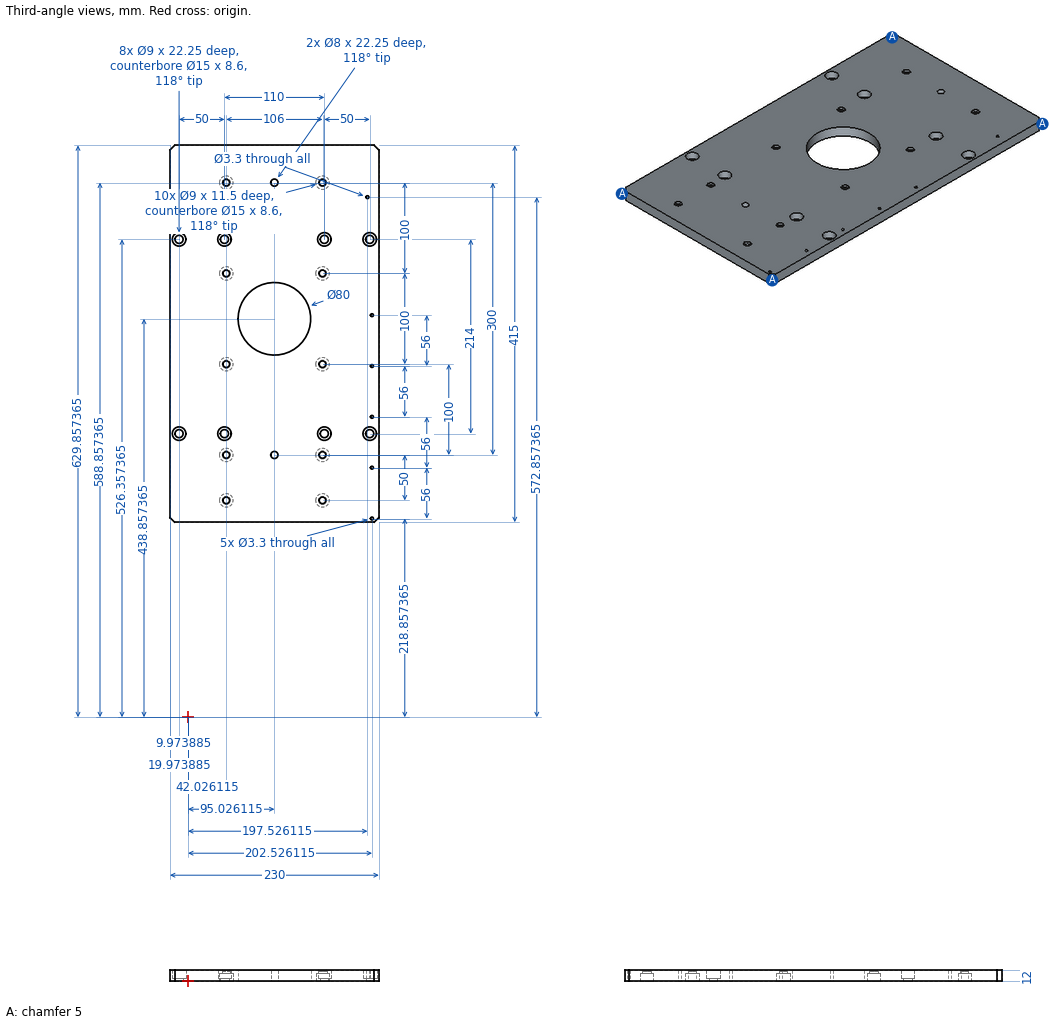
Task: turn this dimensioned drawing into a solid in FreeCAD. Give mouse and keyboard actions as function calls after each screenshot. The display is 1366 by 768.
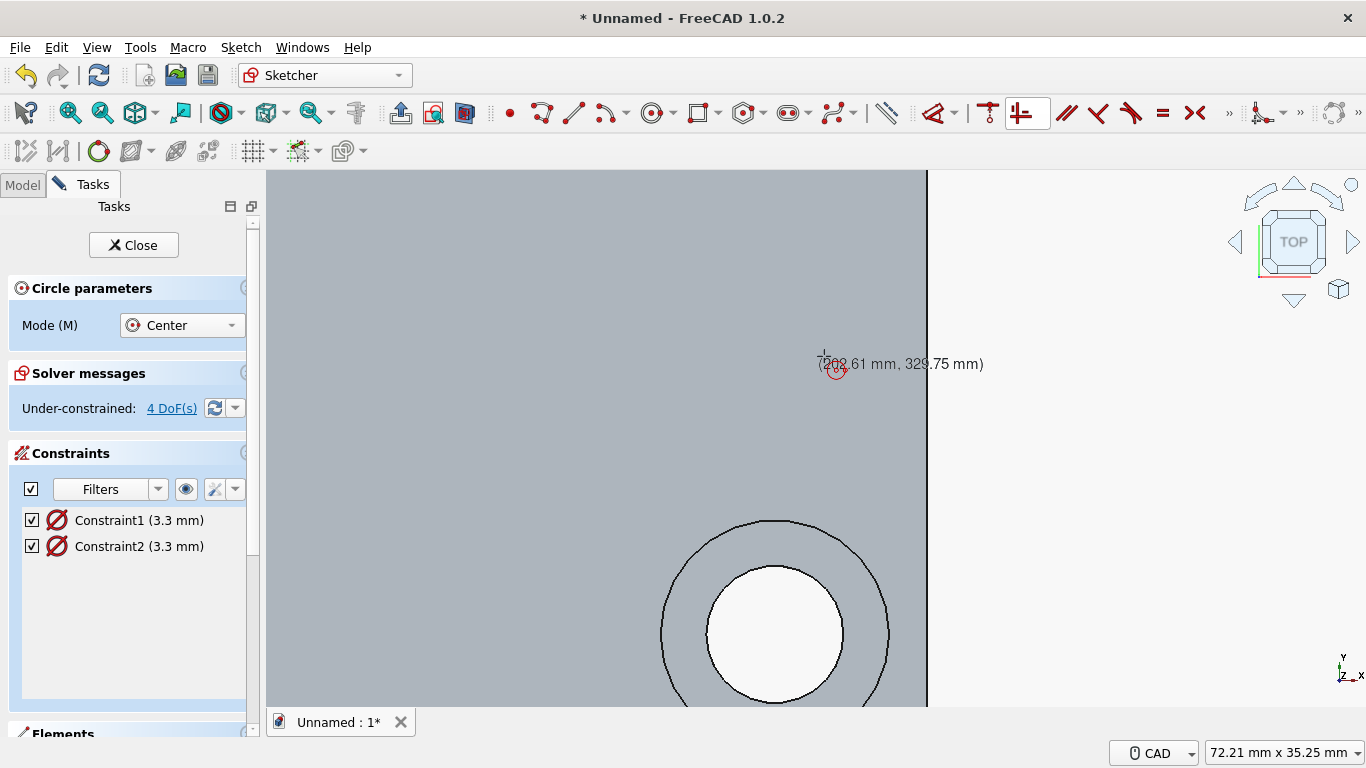
scroll(824, 356, down, 15)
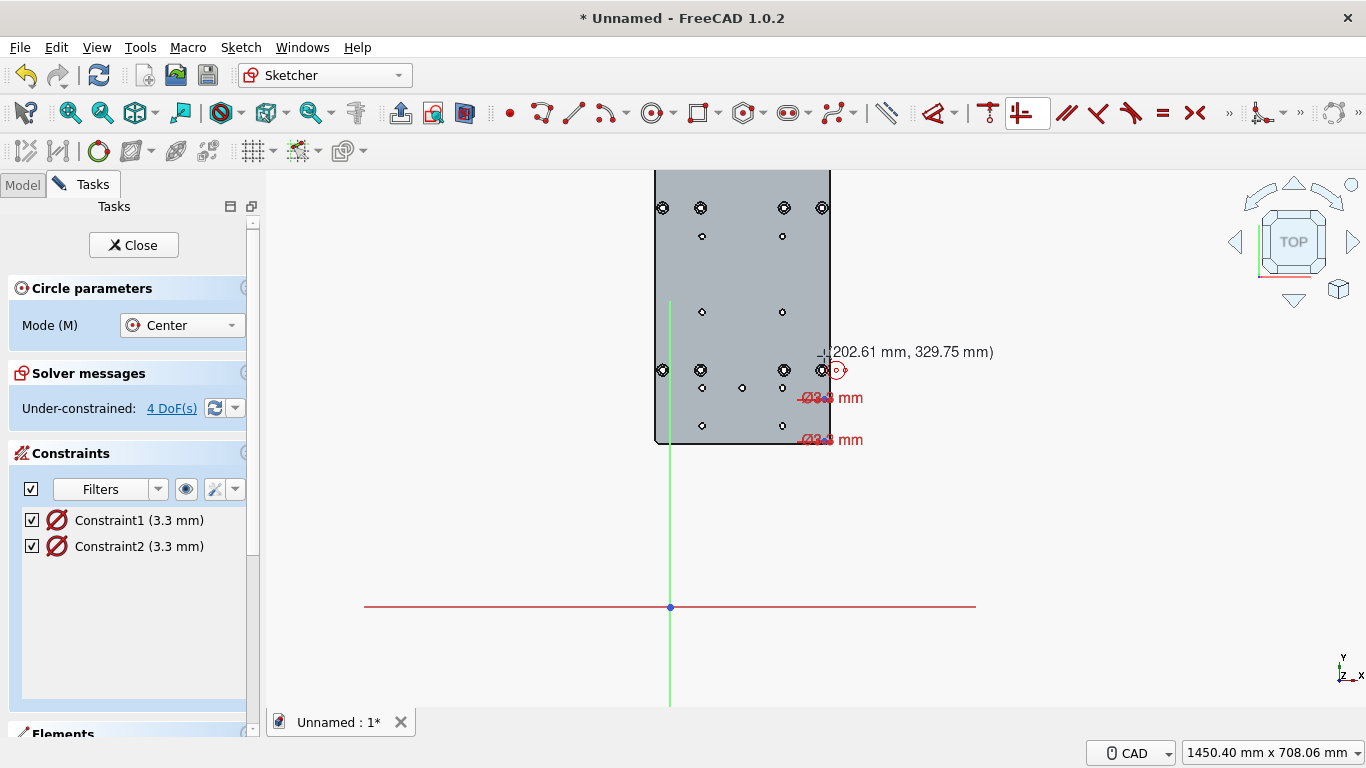
click(824, 356)
move(825, 355)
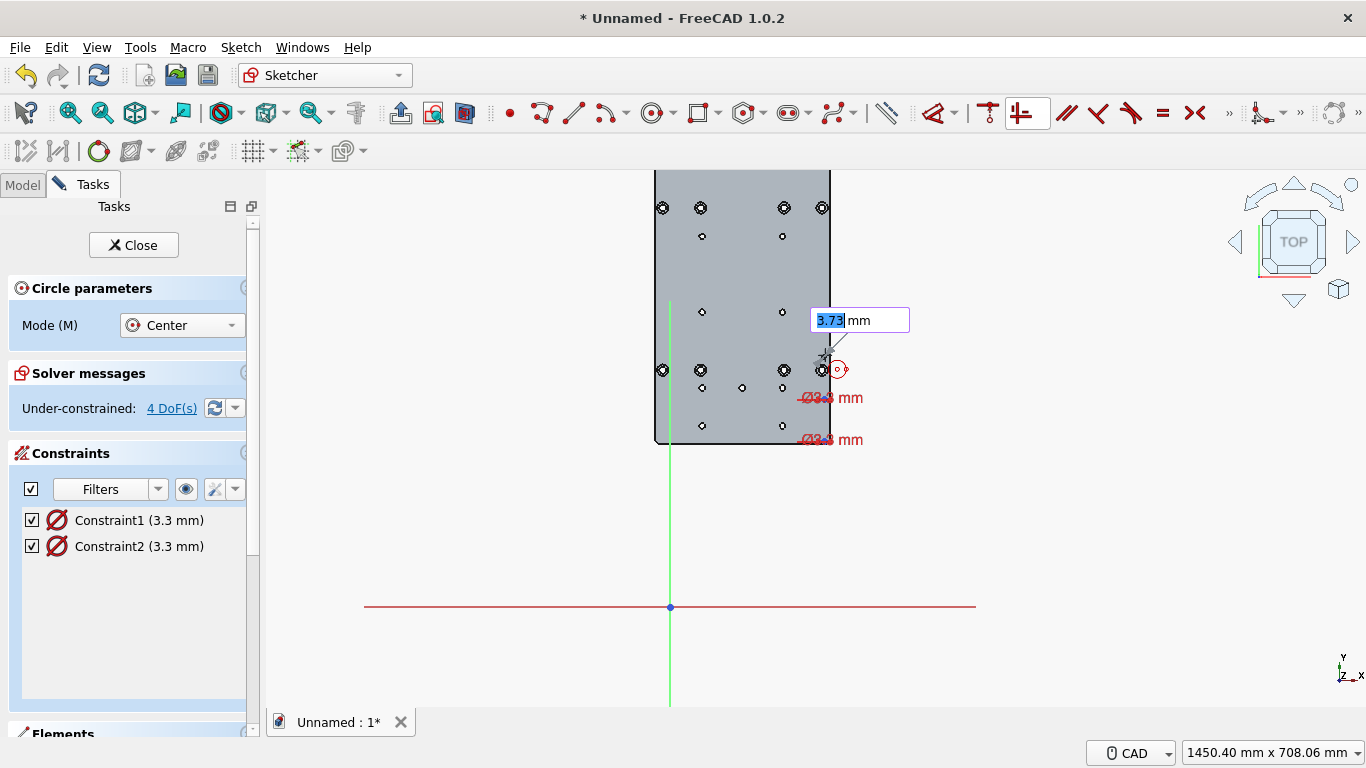
text(3.3)
key(Return)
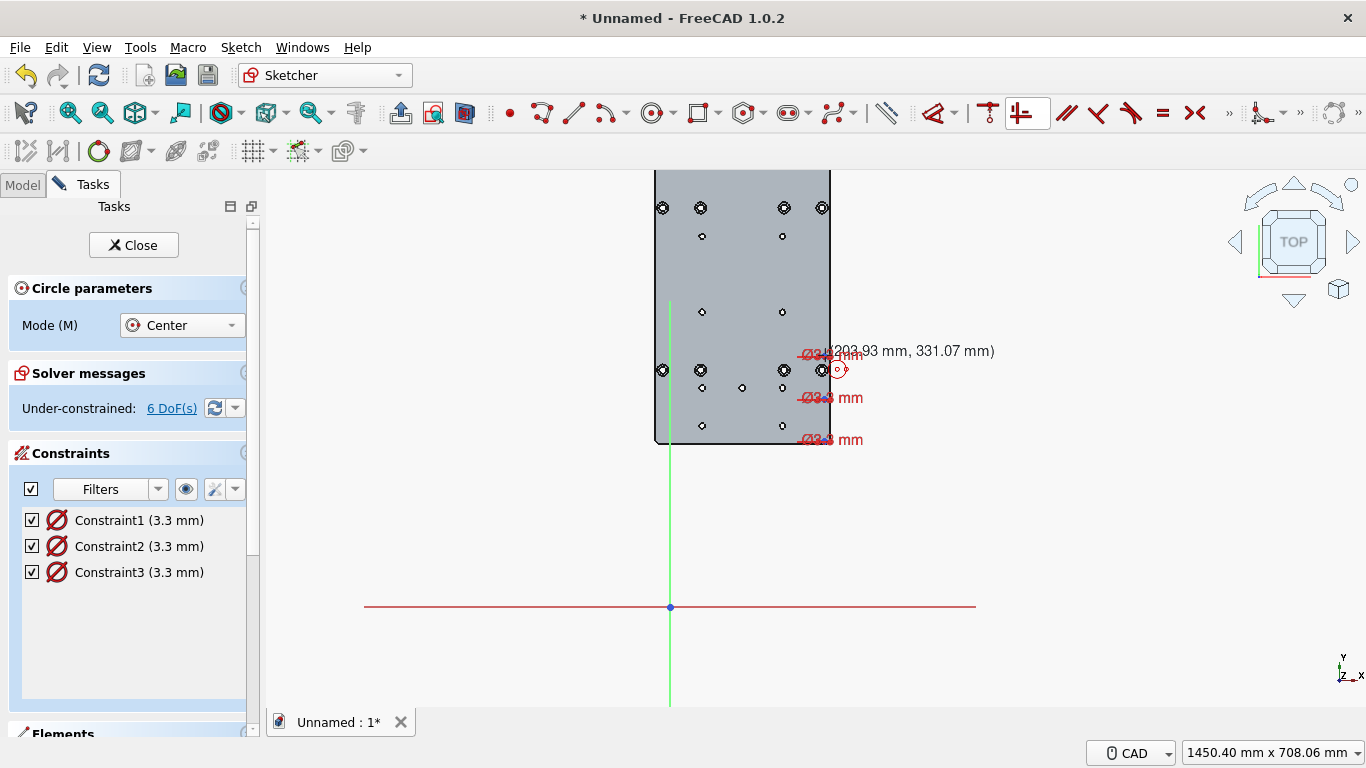
scroll(824, 314, up, 15)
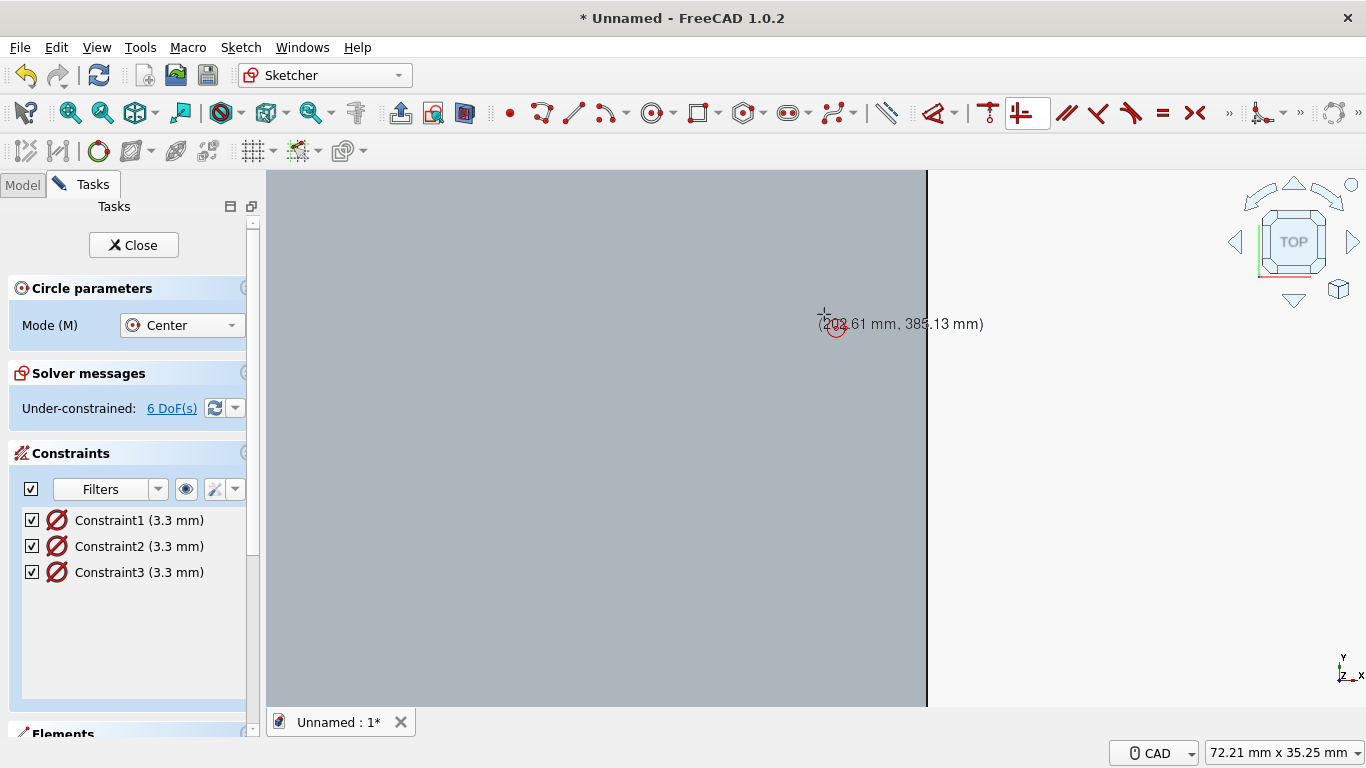
scroll(824, 314, down, 15)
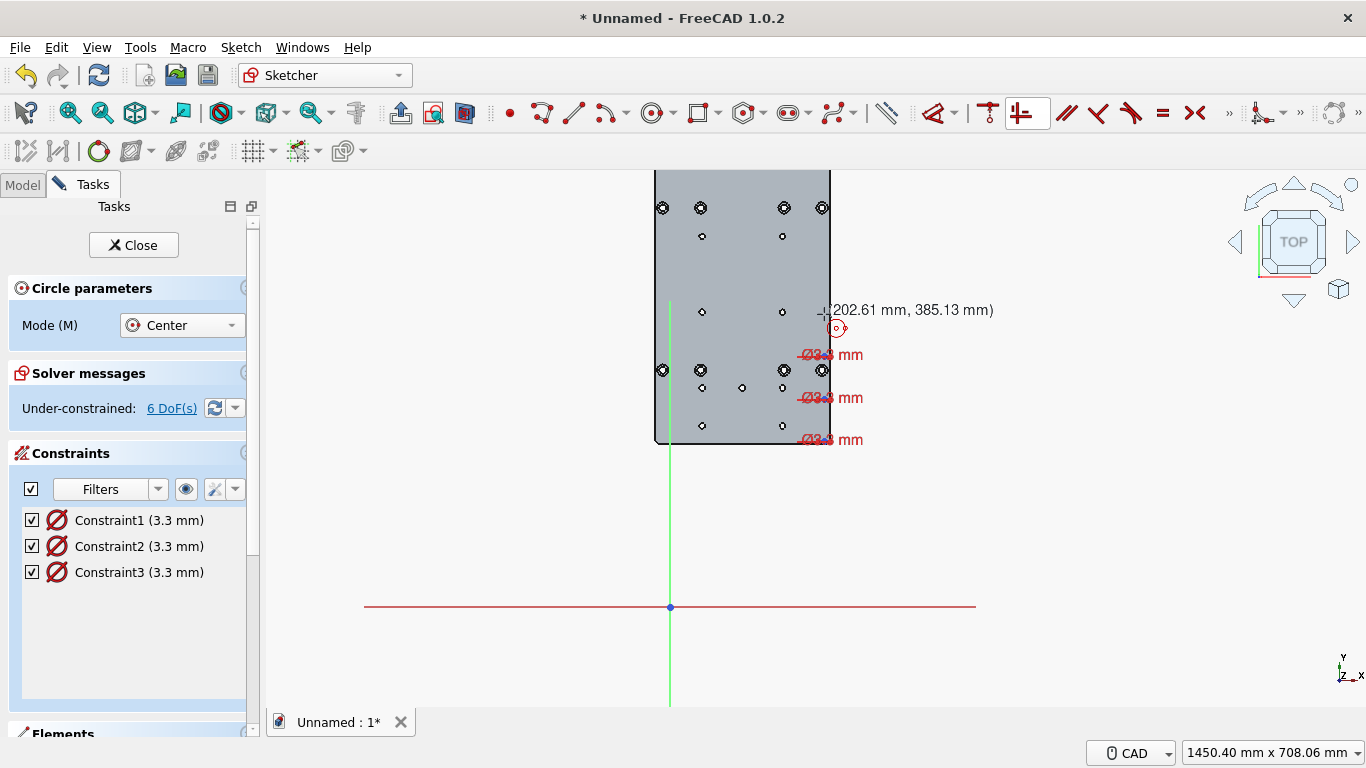
click(824, 314)
move(825, 313)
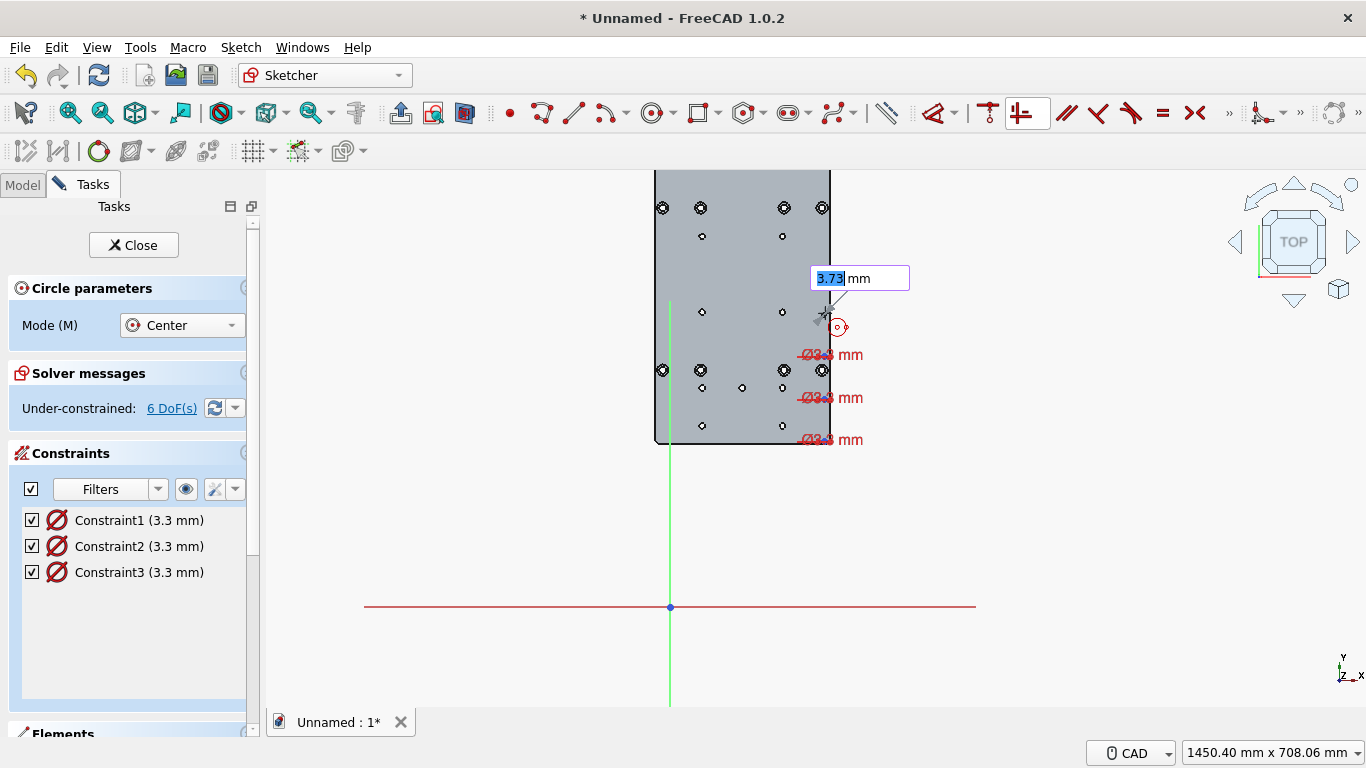
text(3.3)
key(Return)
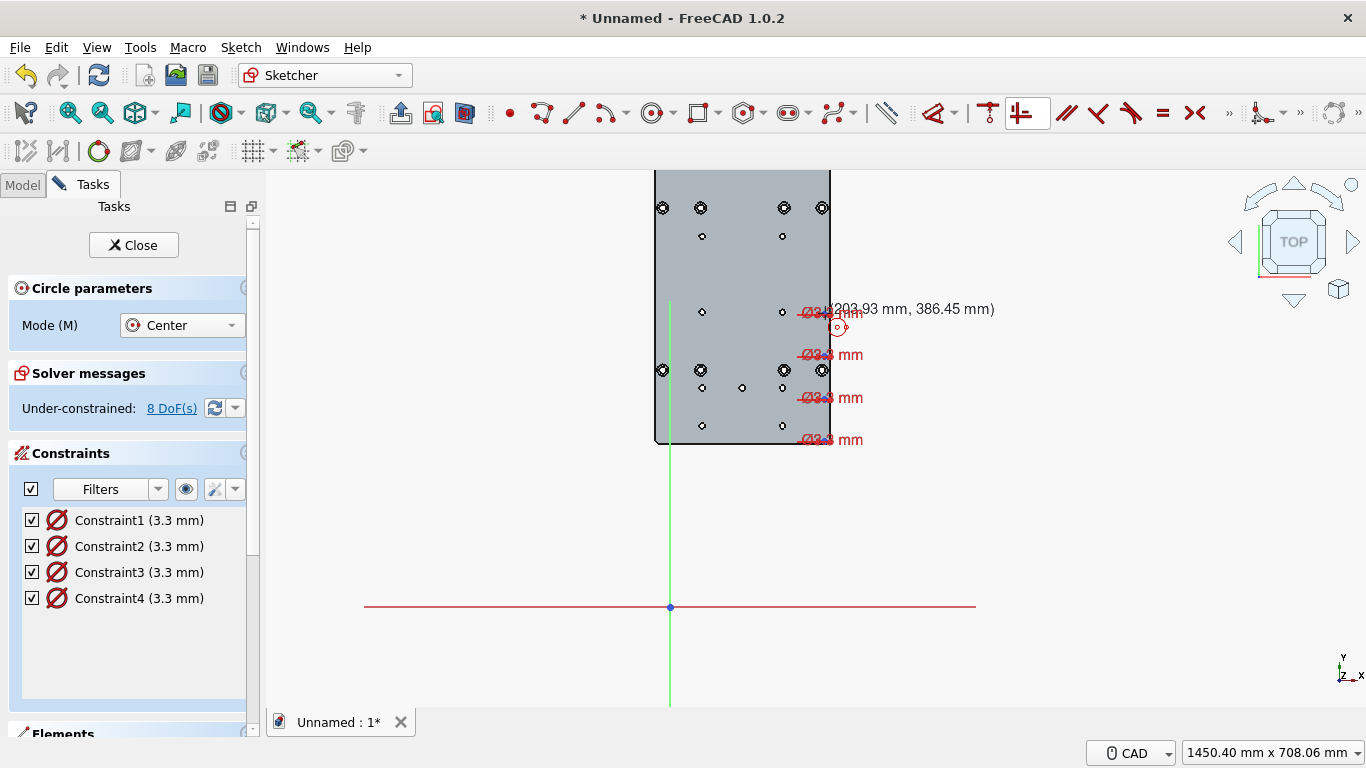
scroll(824, 271, up, 15)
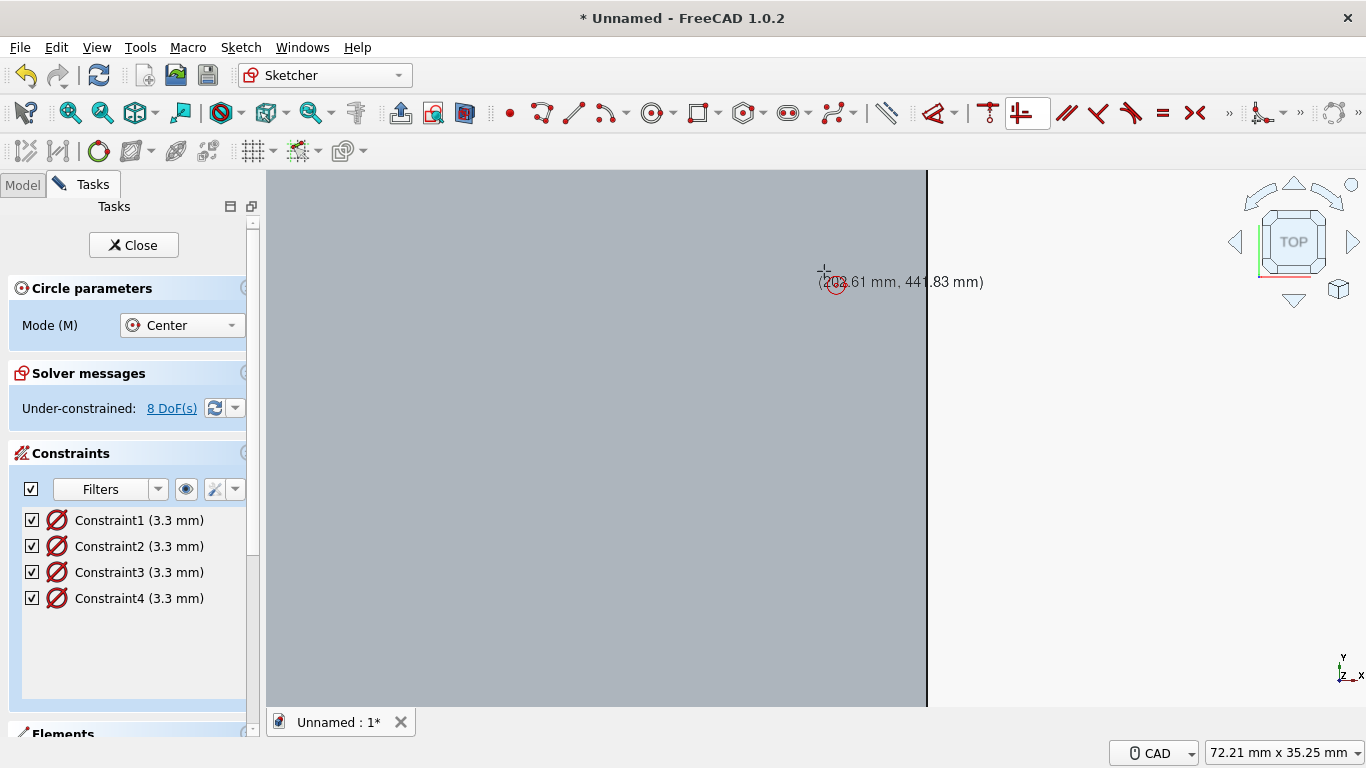
scroll(824, 271, down, 15)